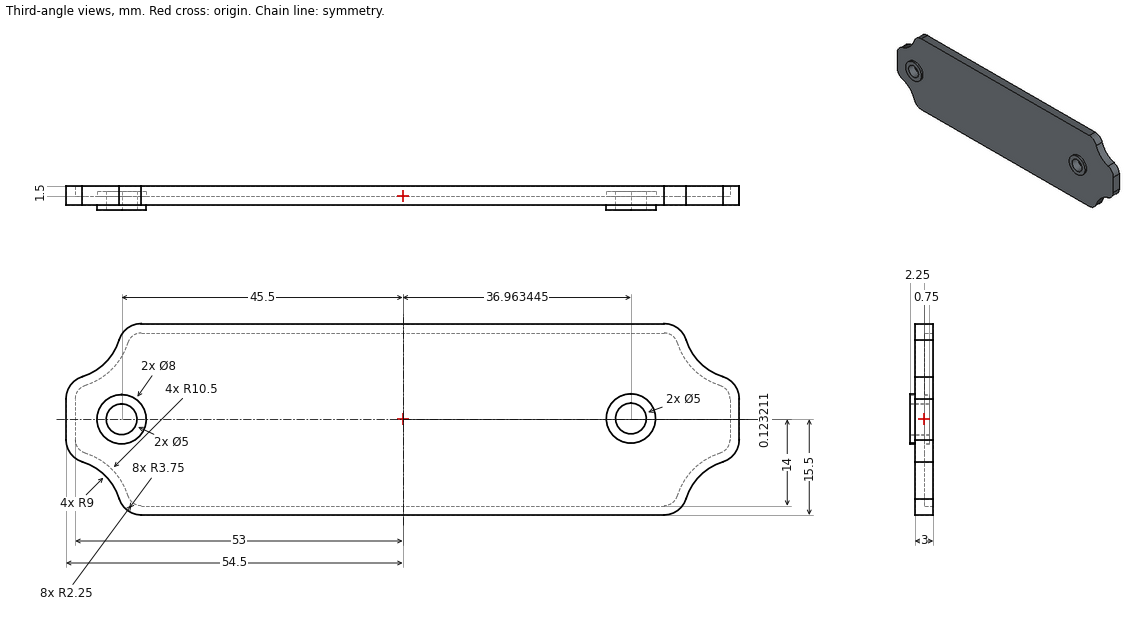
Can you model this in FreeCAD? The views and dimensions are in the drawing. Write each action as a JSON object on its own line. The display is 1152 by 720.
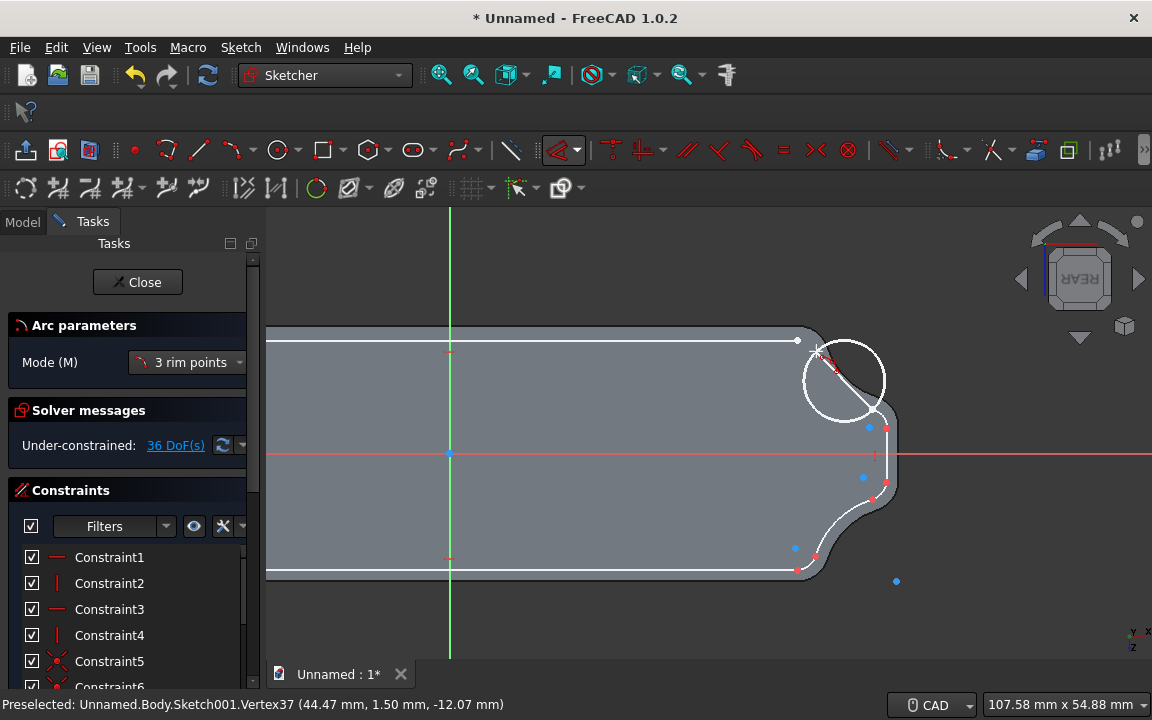
{"action": "scroll", "coordinate": [837, 387], "scroll_direction": "up", "scroll_amount": 3}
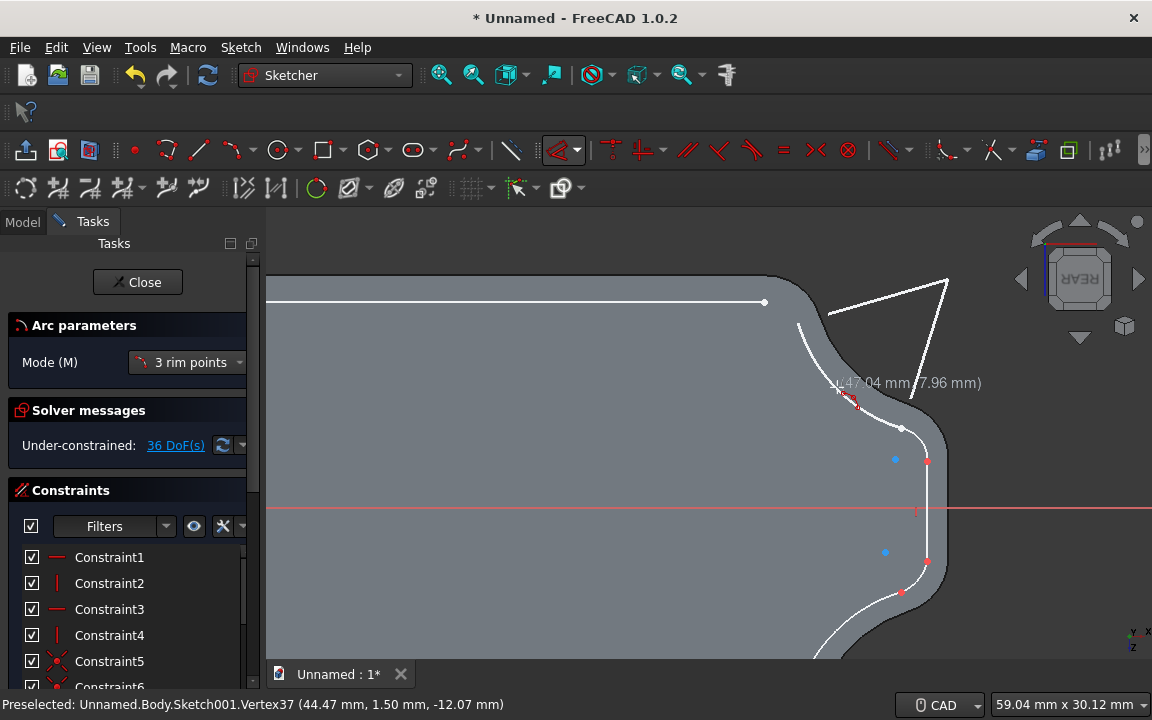
{"action": "left_click", "coordinate": [837, 387]}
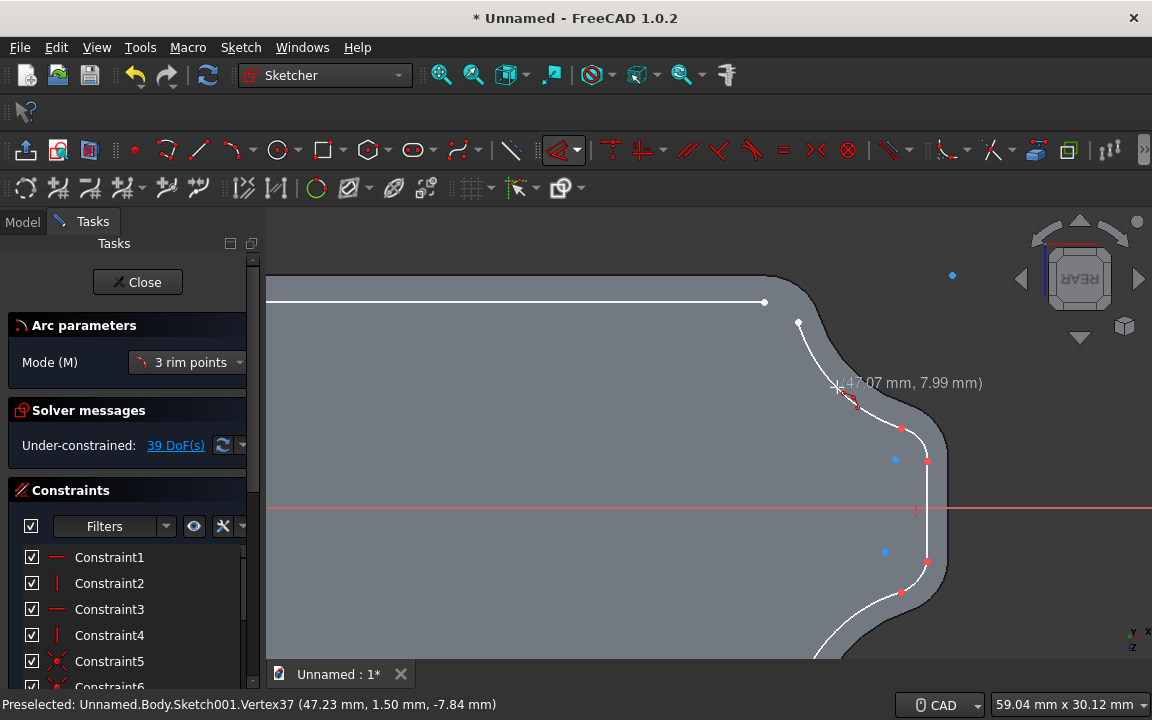
{"action": "left_click", "coordinate": [798, 323]}
{"action": "left_click", "coordinate": [765, 302]}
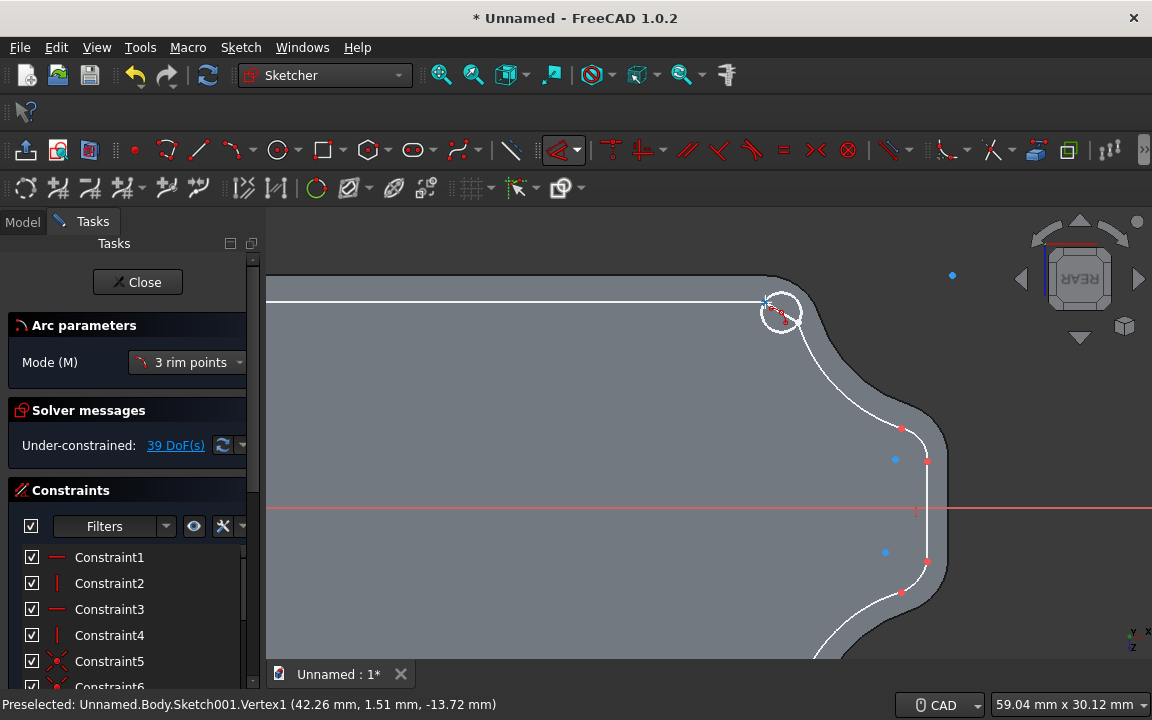
{"action": "scroll", "coordinate": [786, 304], "scroll_direction": "up", "scroll_amount": 5}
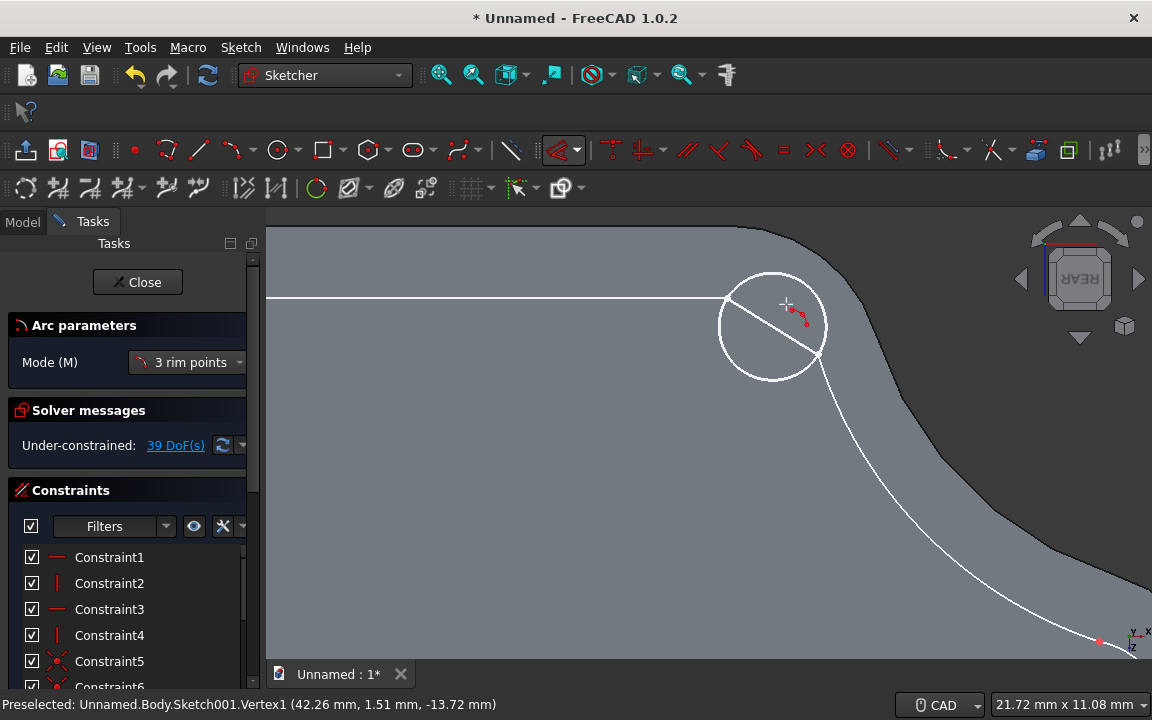
{"action": "left_click", "coordinate": [784, 305]}
{"action": "key", "text": "Escape"}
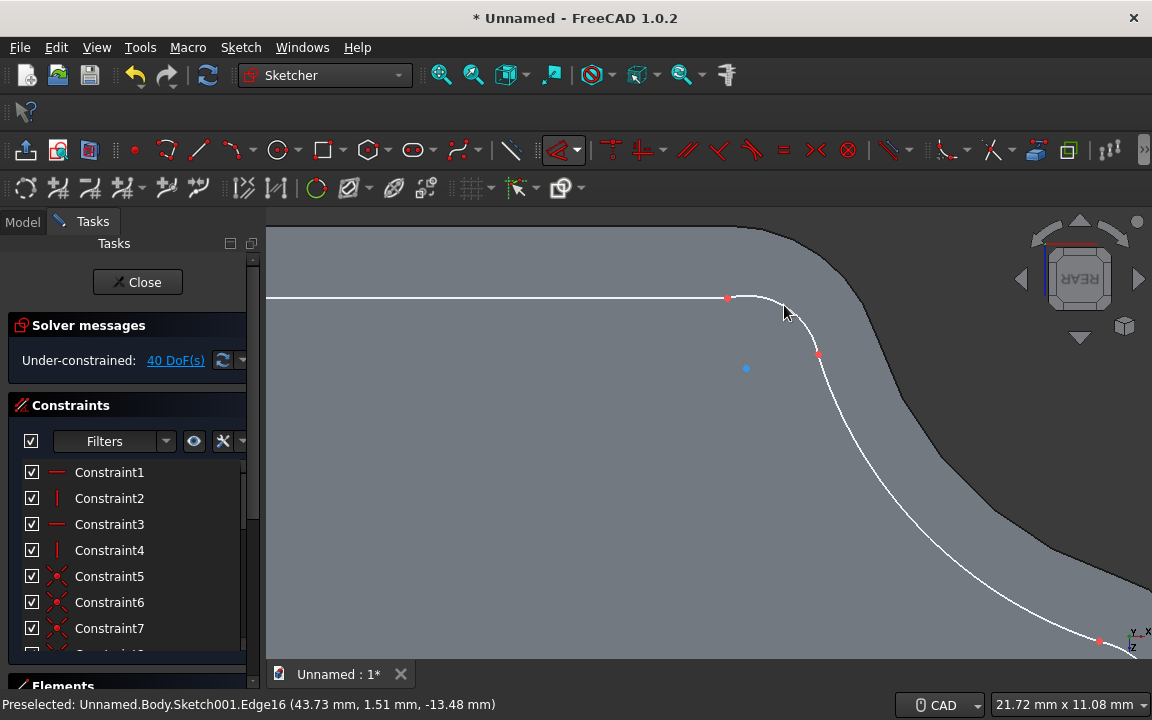
{"action": "scroll", "coordinate": [845, 380], "scroll_direction": "down", "scroll_amount": 11}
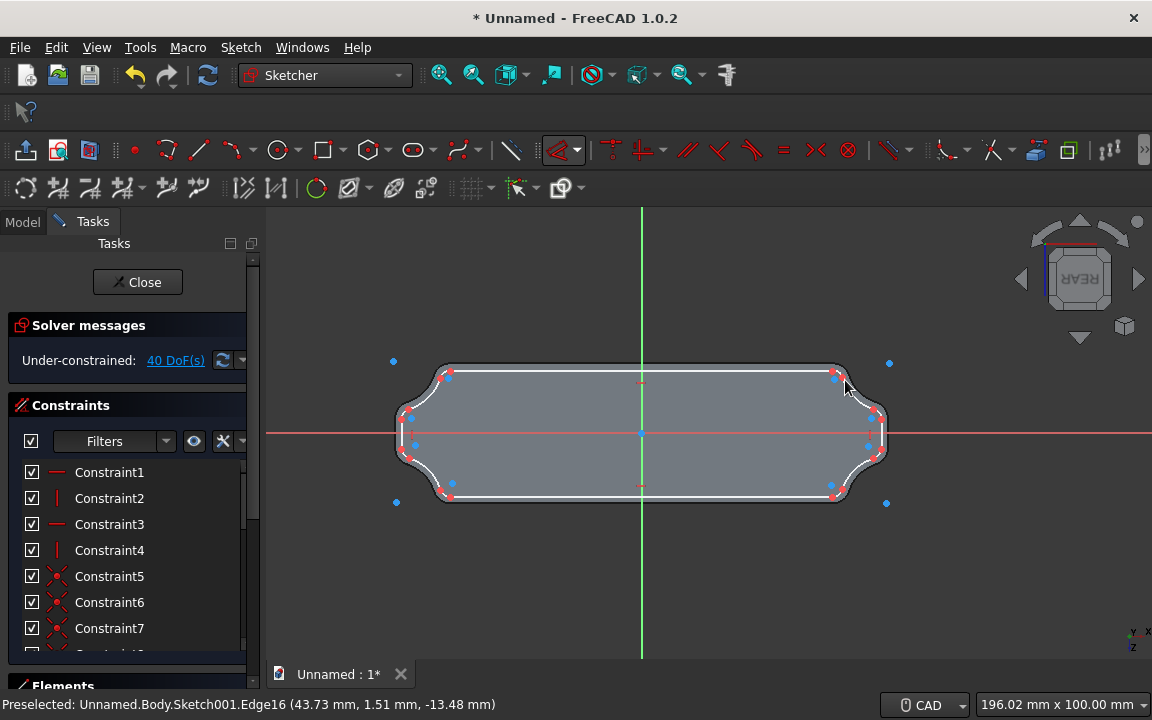
{"action": "left_click", "coordinate": [718, 371]}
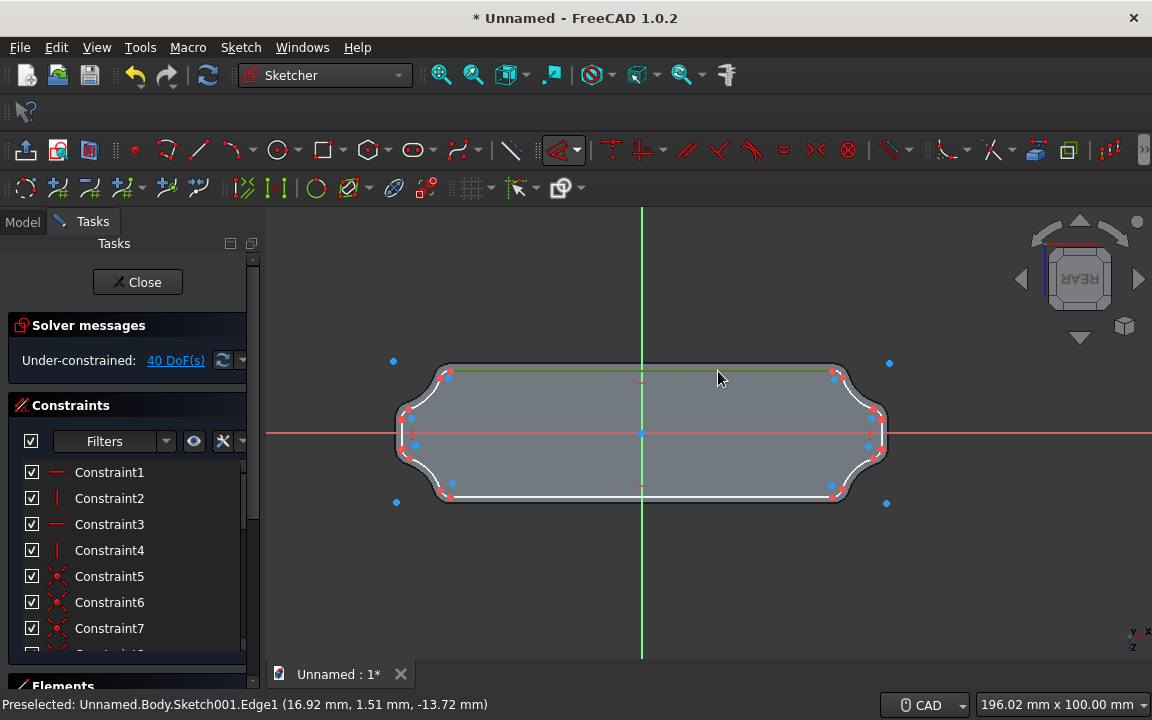
{"action": "scroll", "coordinate": [444, 372], "scroll_direction": "up", "scroll_amount": 4}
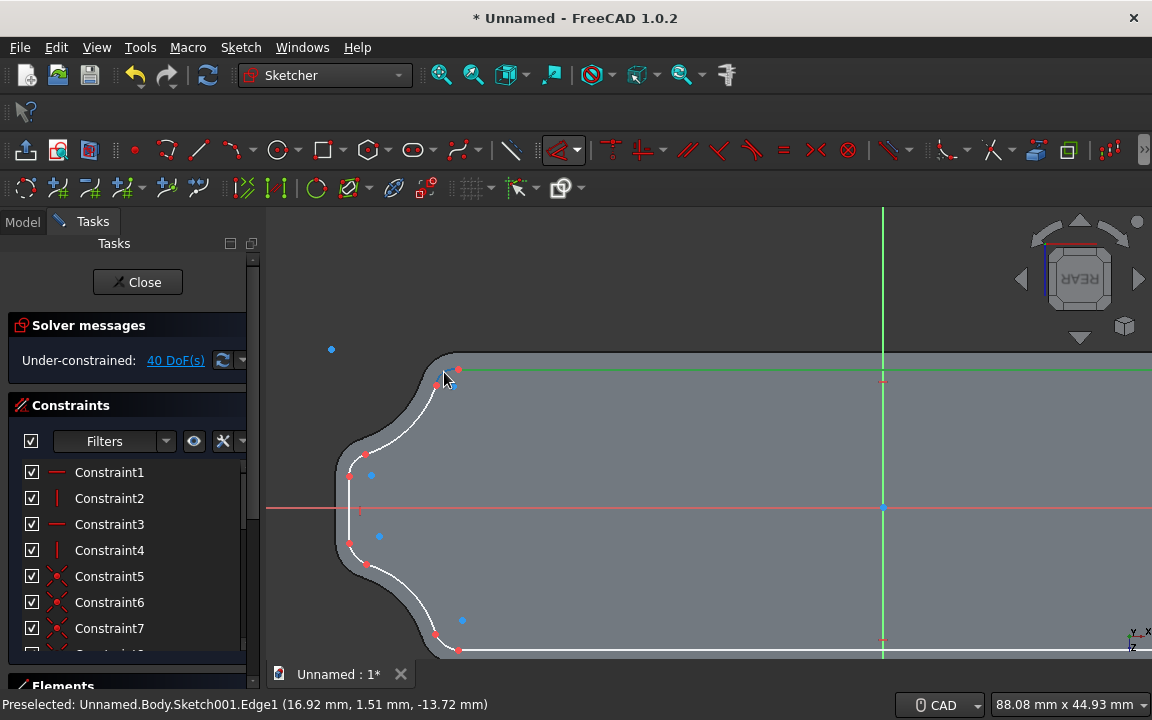
{"action": "left_click", "coordinate": [444, 372]}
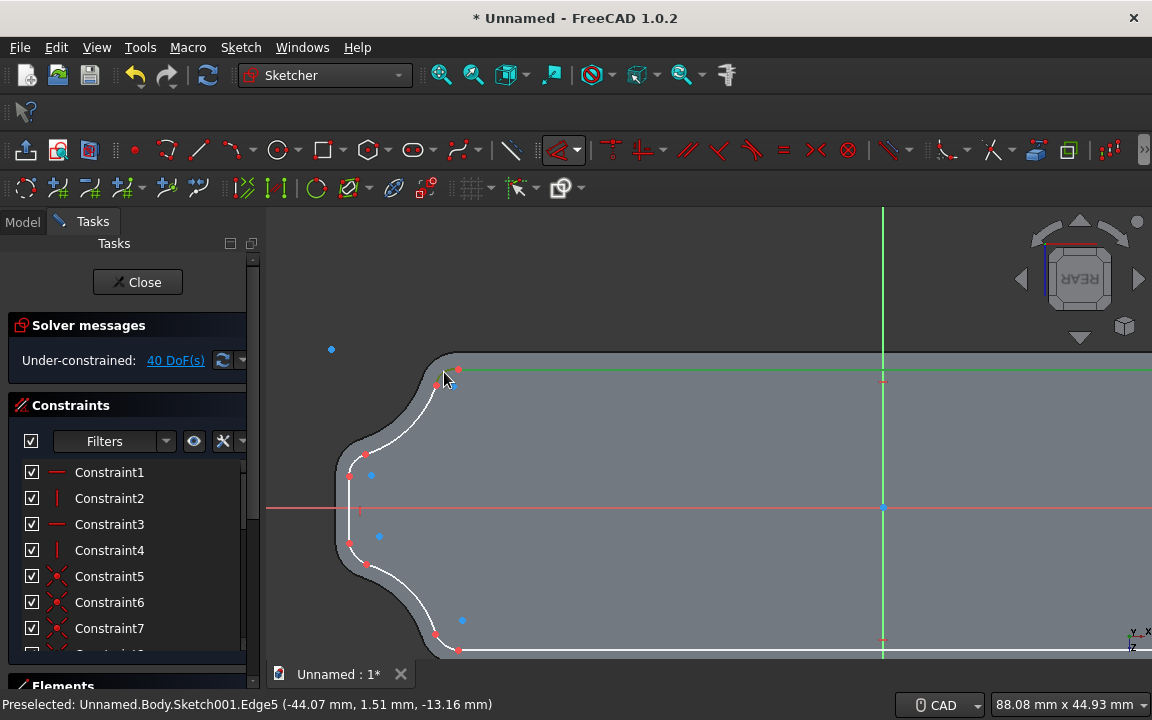
{"action": "left_click", "coordinate": [752, 150]}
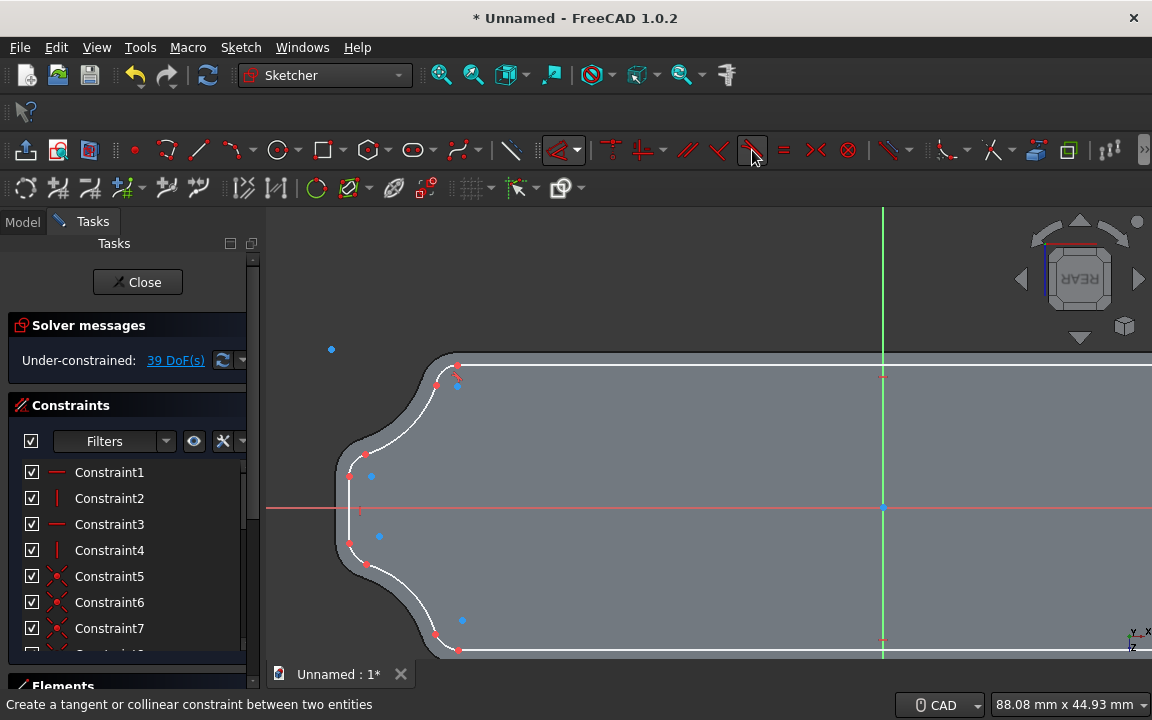
{"action": "left_click", "coordinate": [713, 365]}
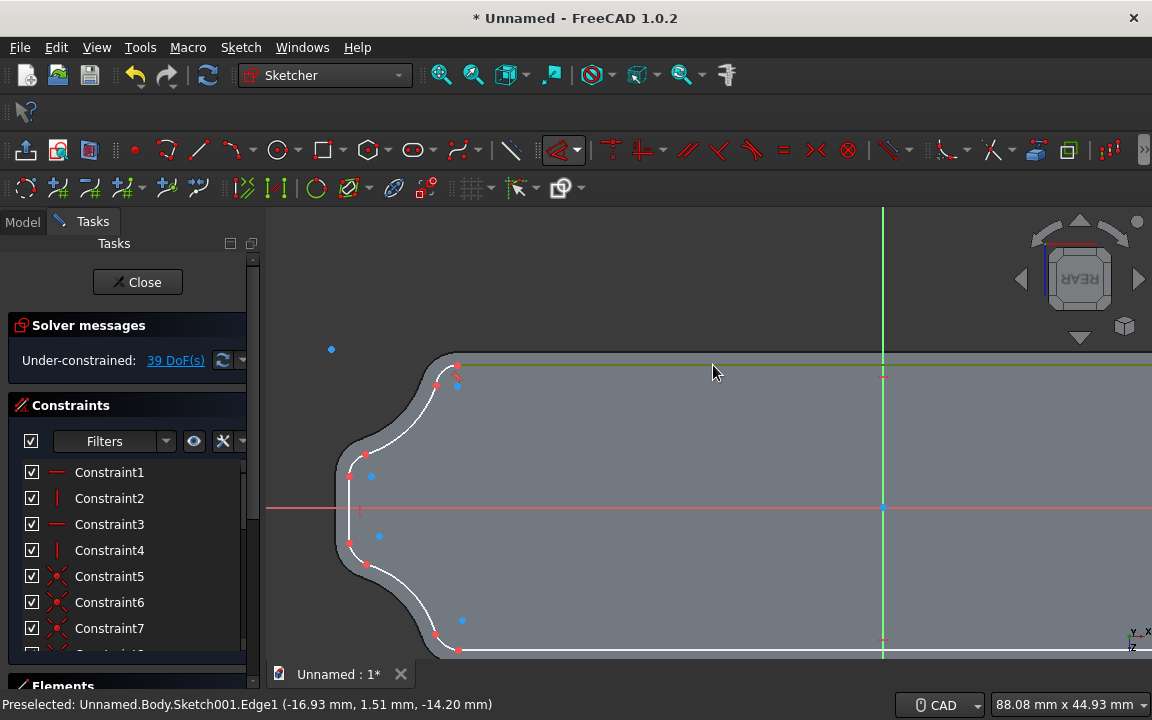
{"action": "scroll", "coordinate": [442, 372], "scroll_direction": "down", "scroll_amount": 4}